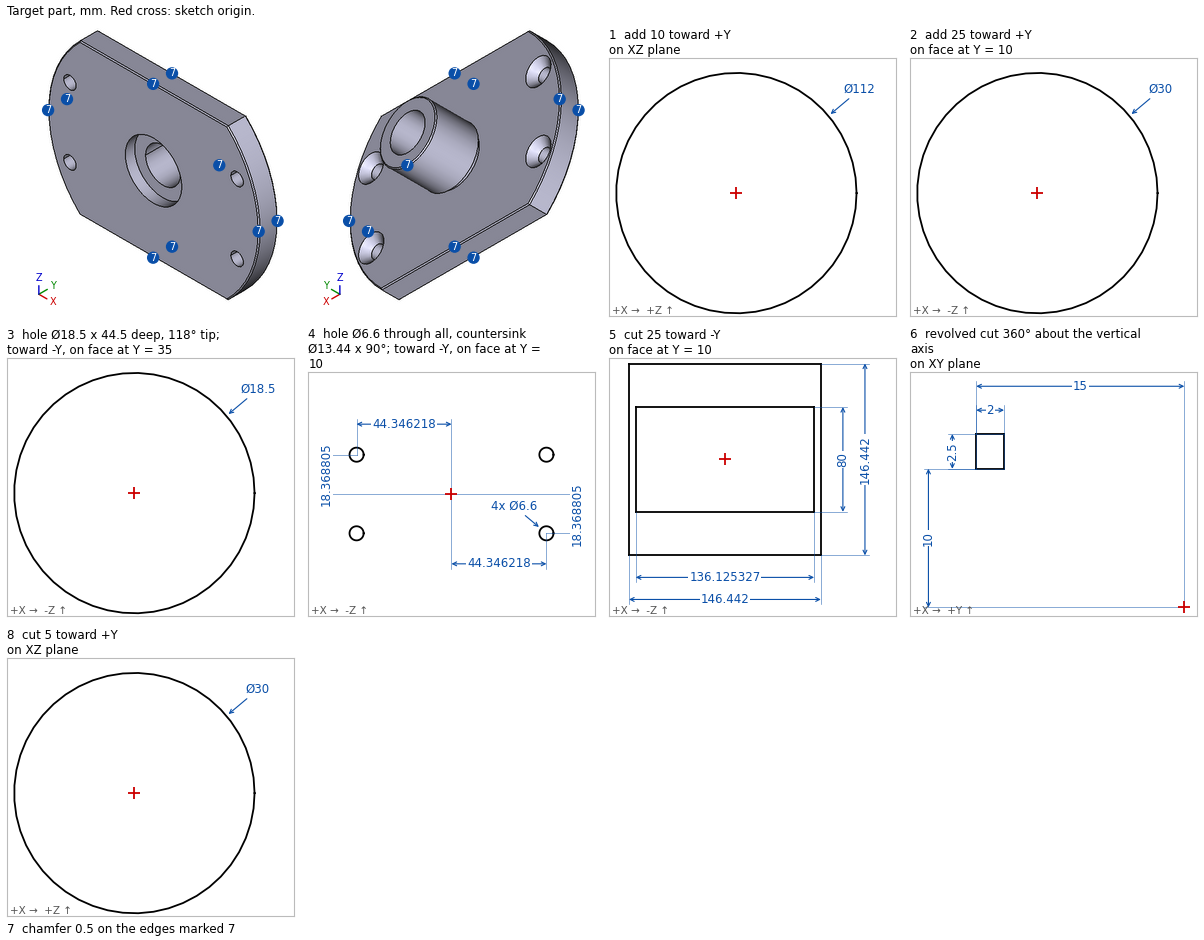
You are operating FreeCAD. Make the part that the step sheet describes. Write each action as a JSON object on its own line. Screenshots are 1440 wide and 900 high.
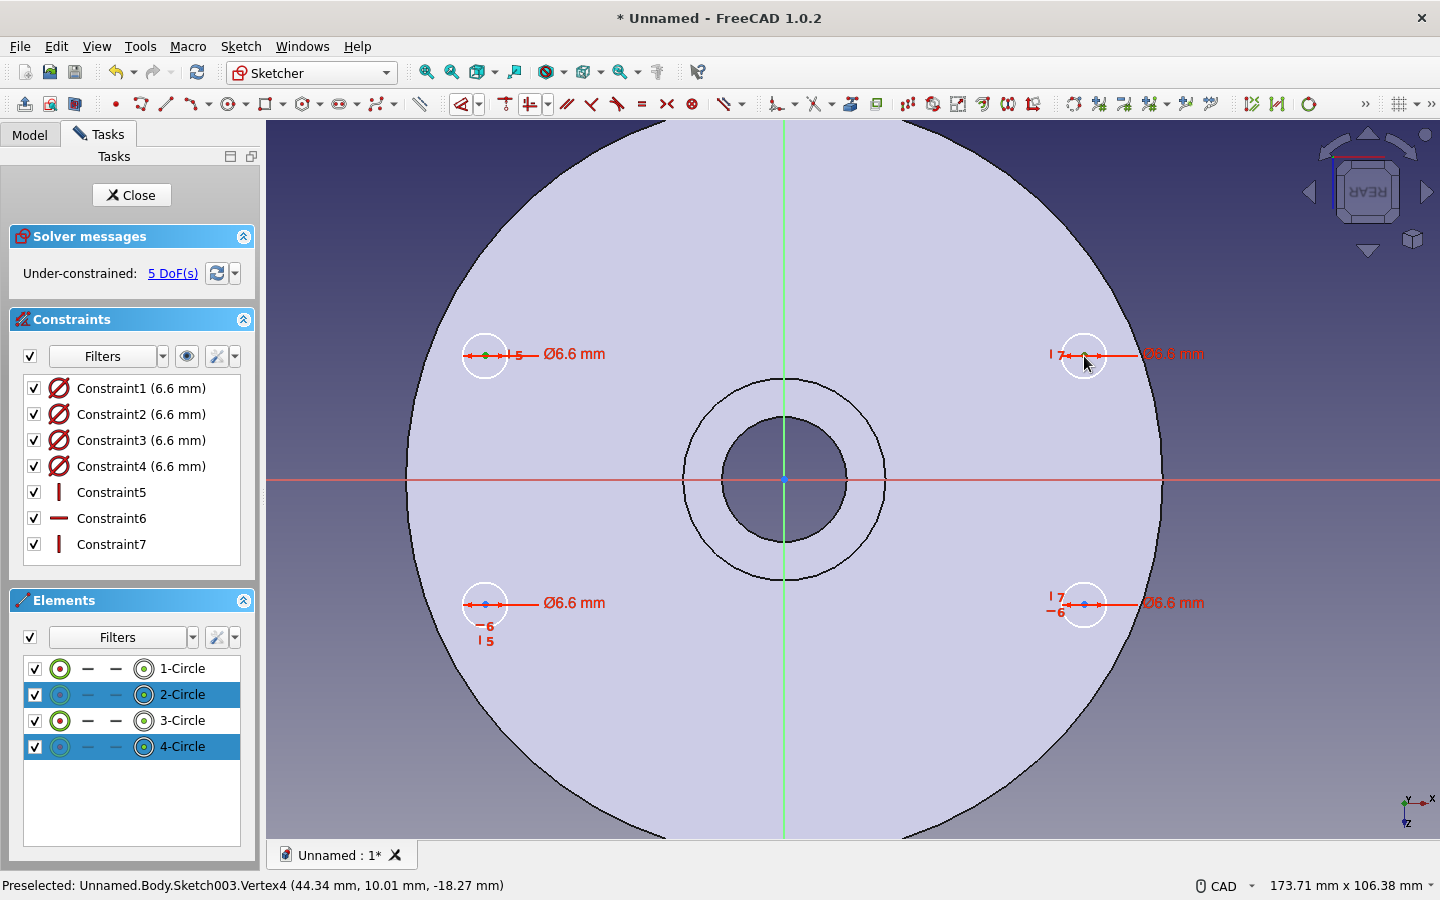
{"action": "key", "text": "h"}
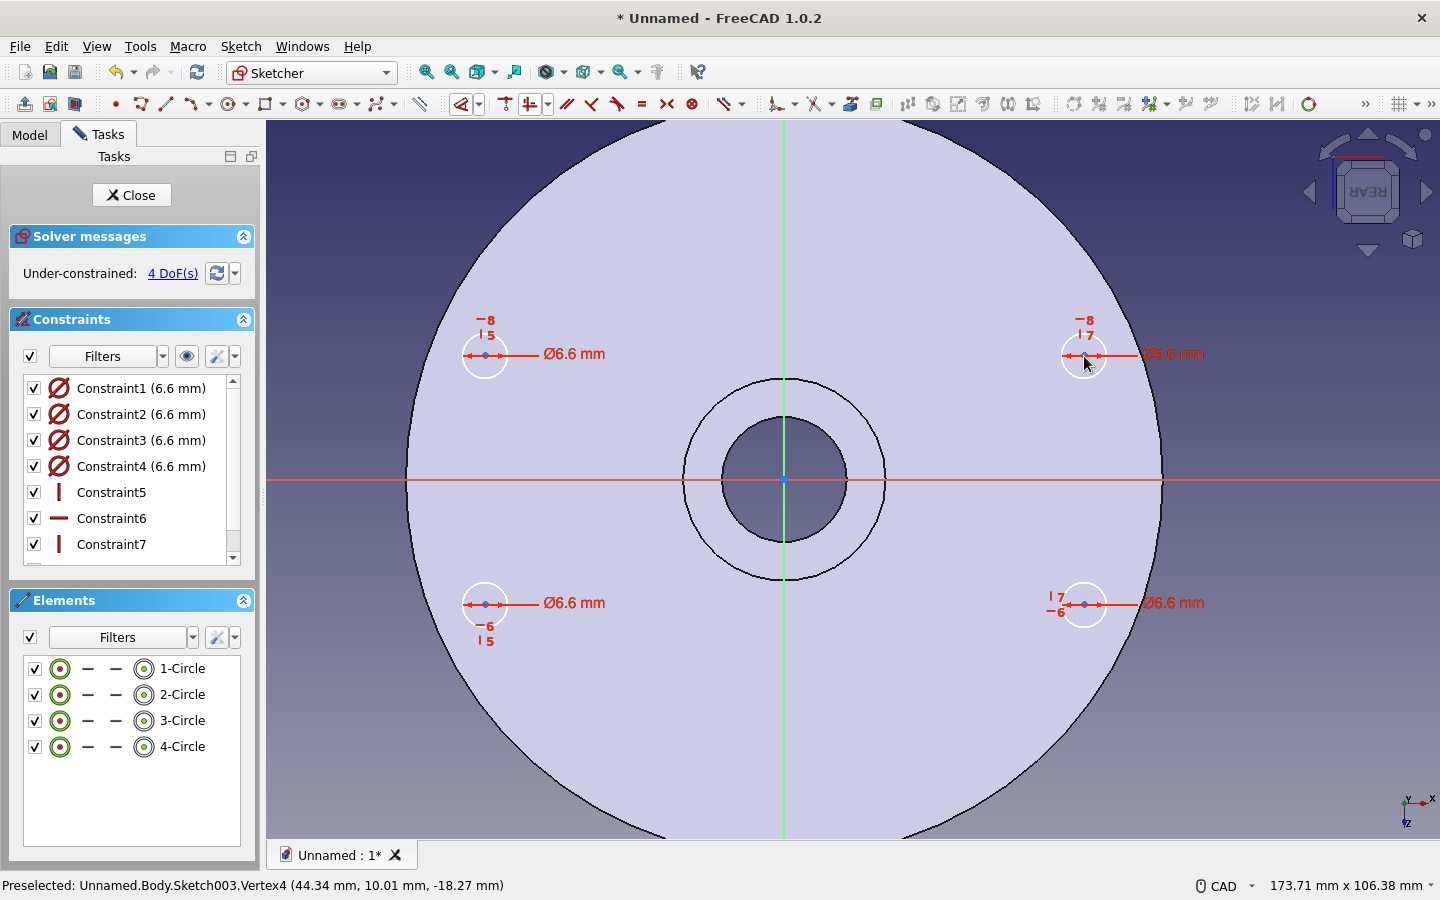
{"action": "left_click", "coordinate": [1084, 605]}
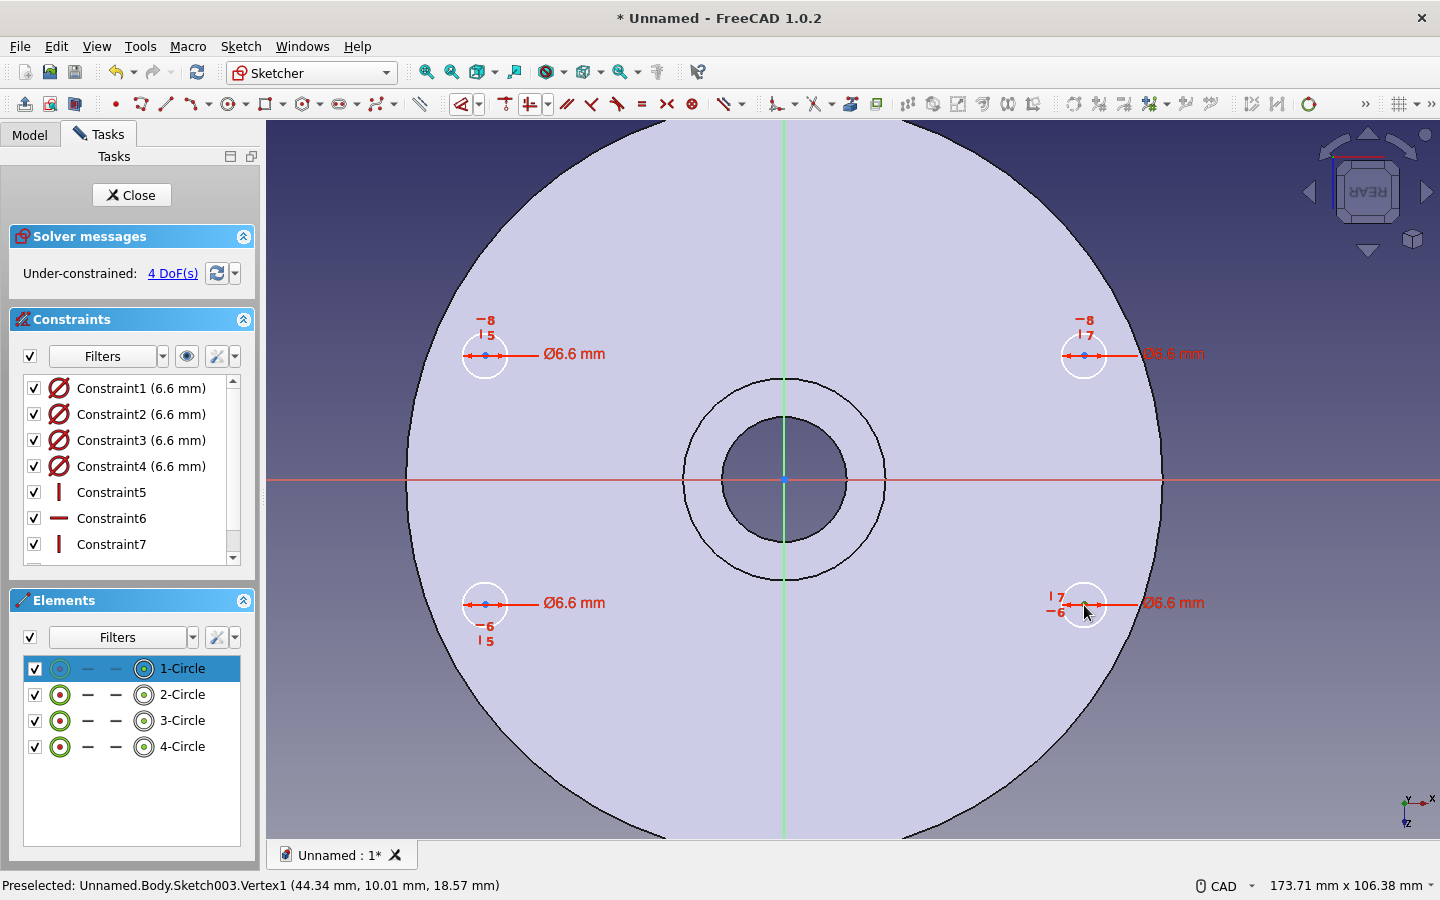
{"action": "key", "text": "l"}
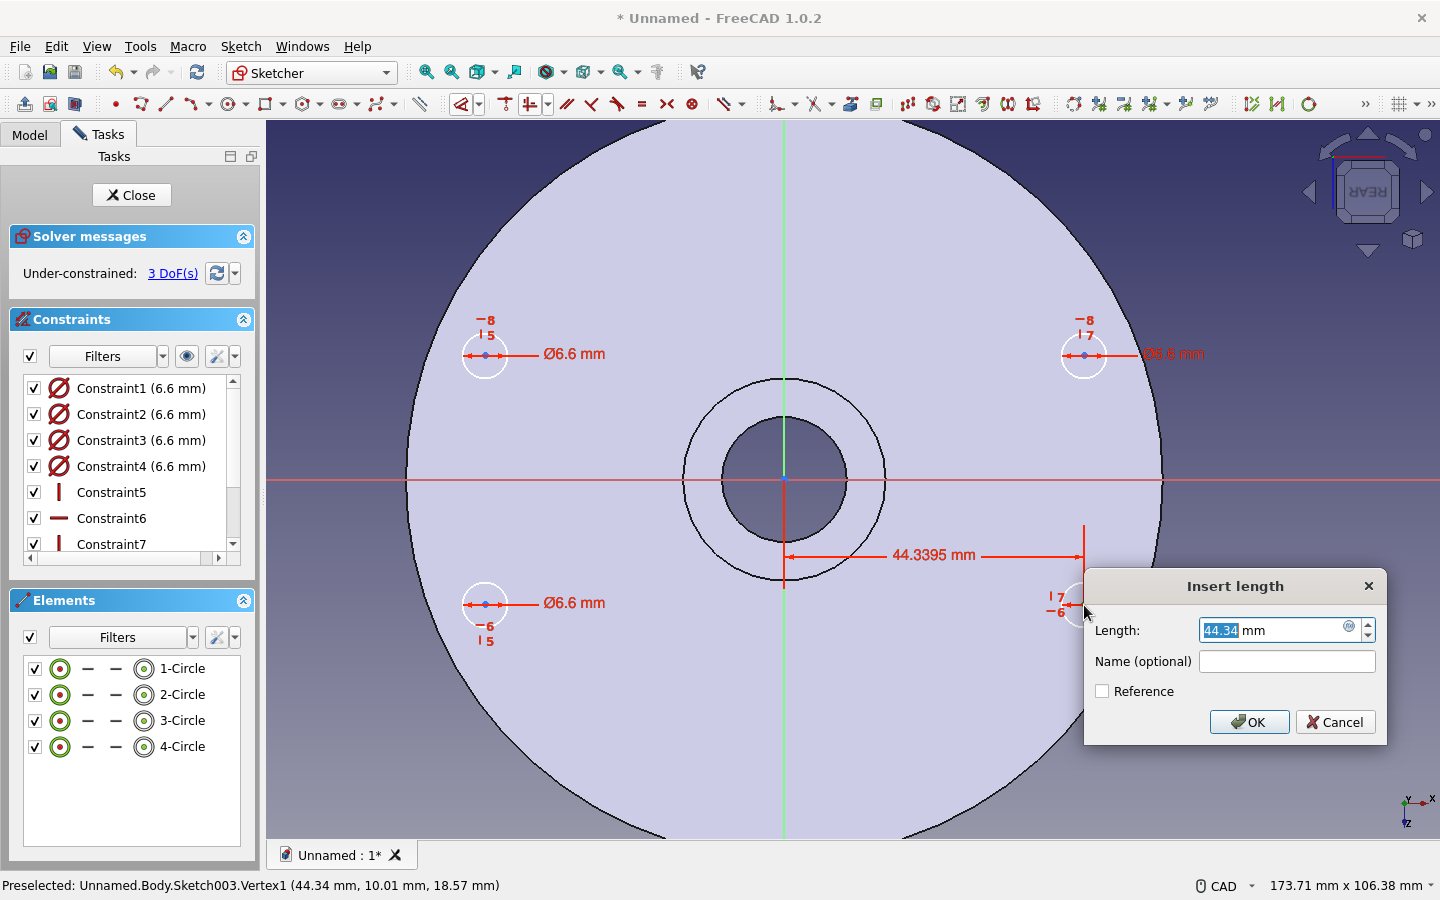
{"action": "type", "text": "44.346218"}
{"action": "key", "text": "Return"}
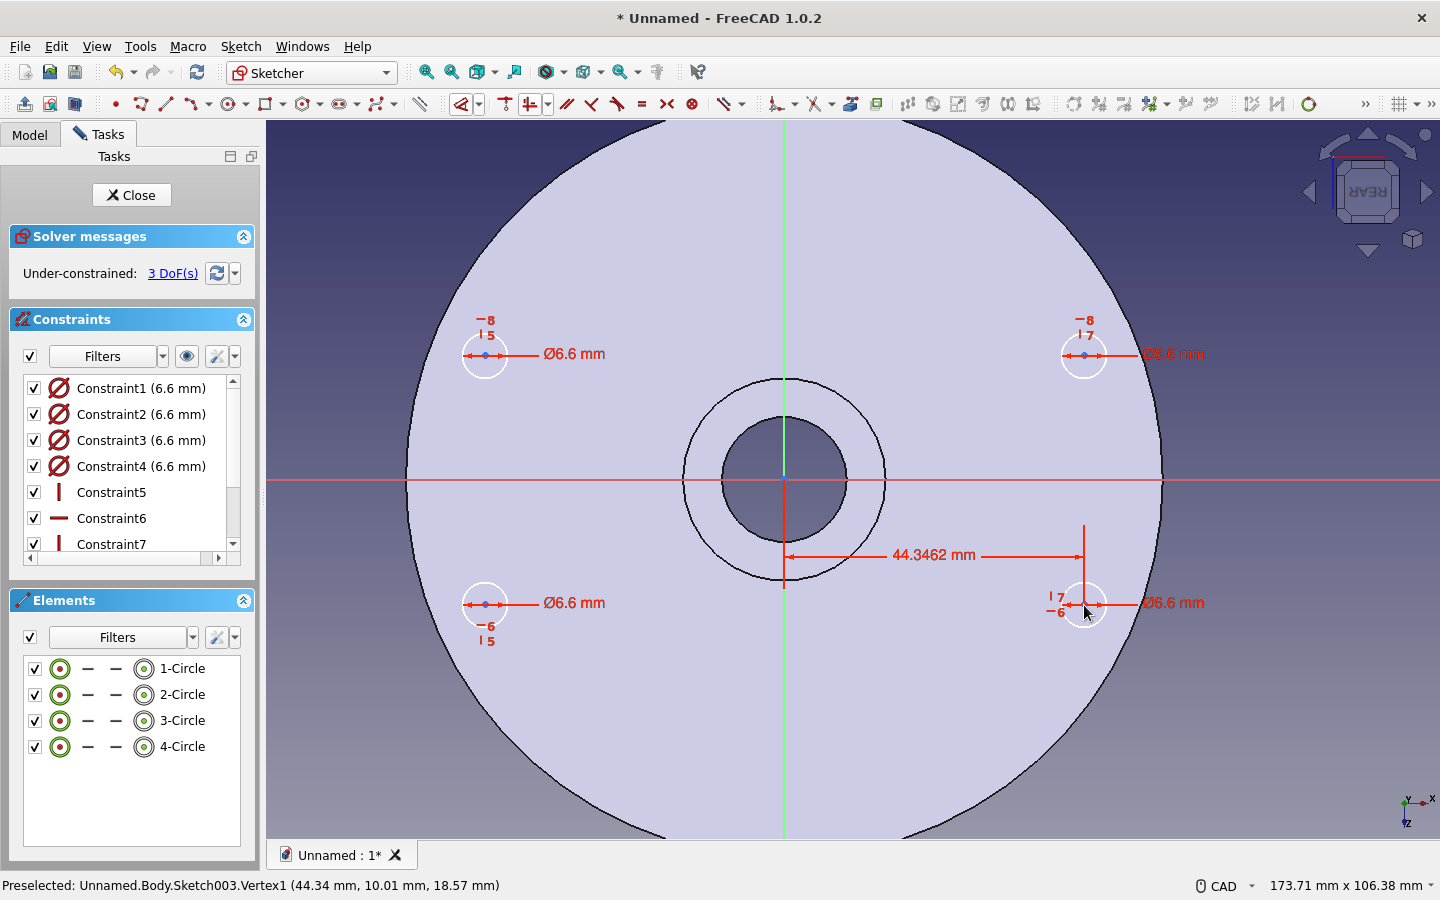
{"action": "left_click", "coordinate": [1084, 605]}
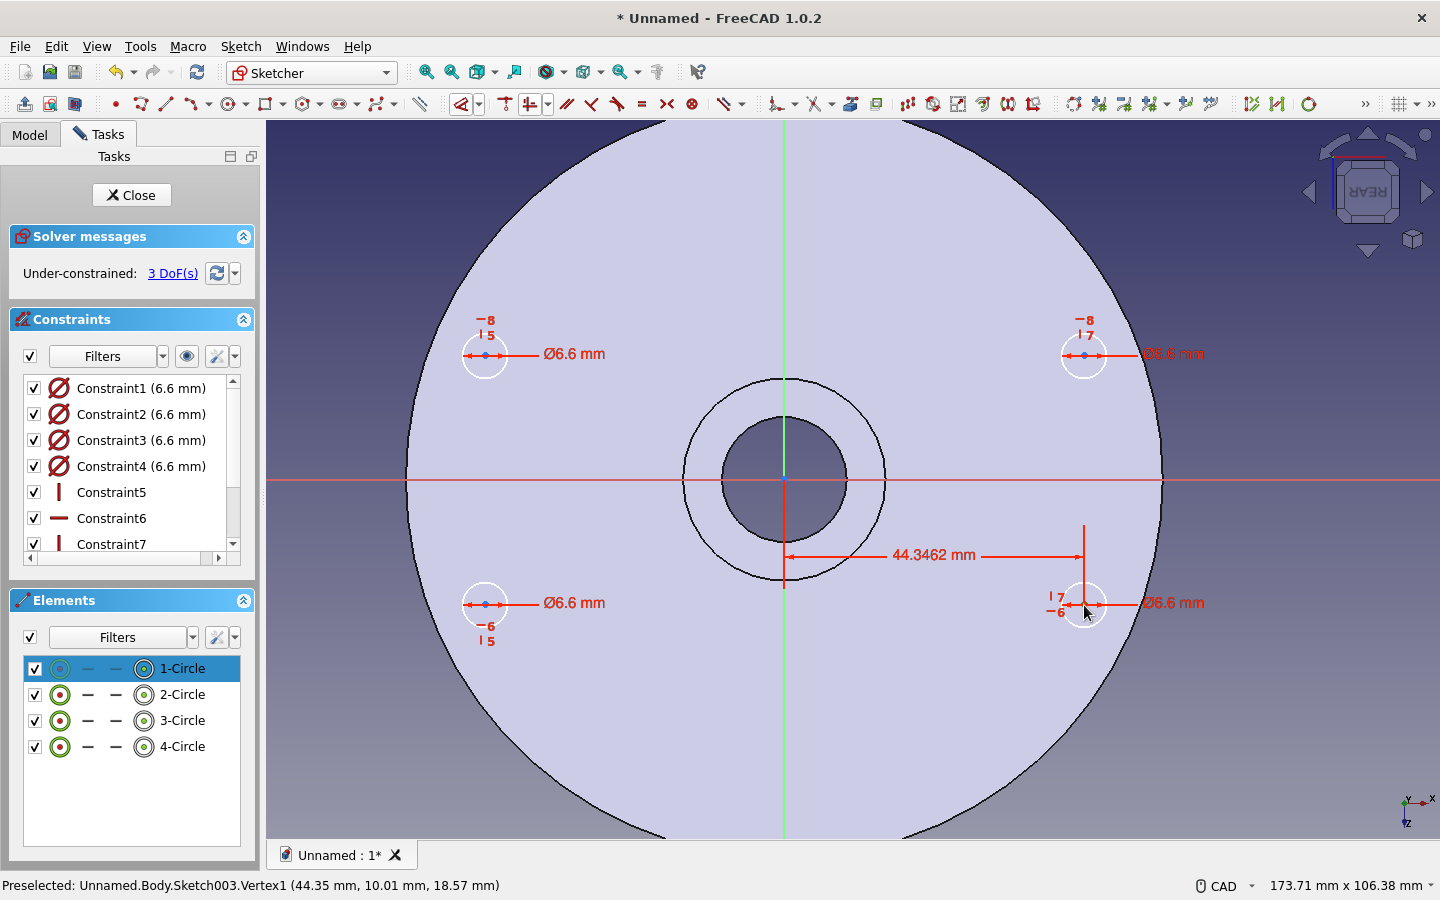
{"action": "key", "text": "i"}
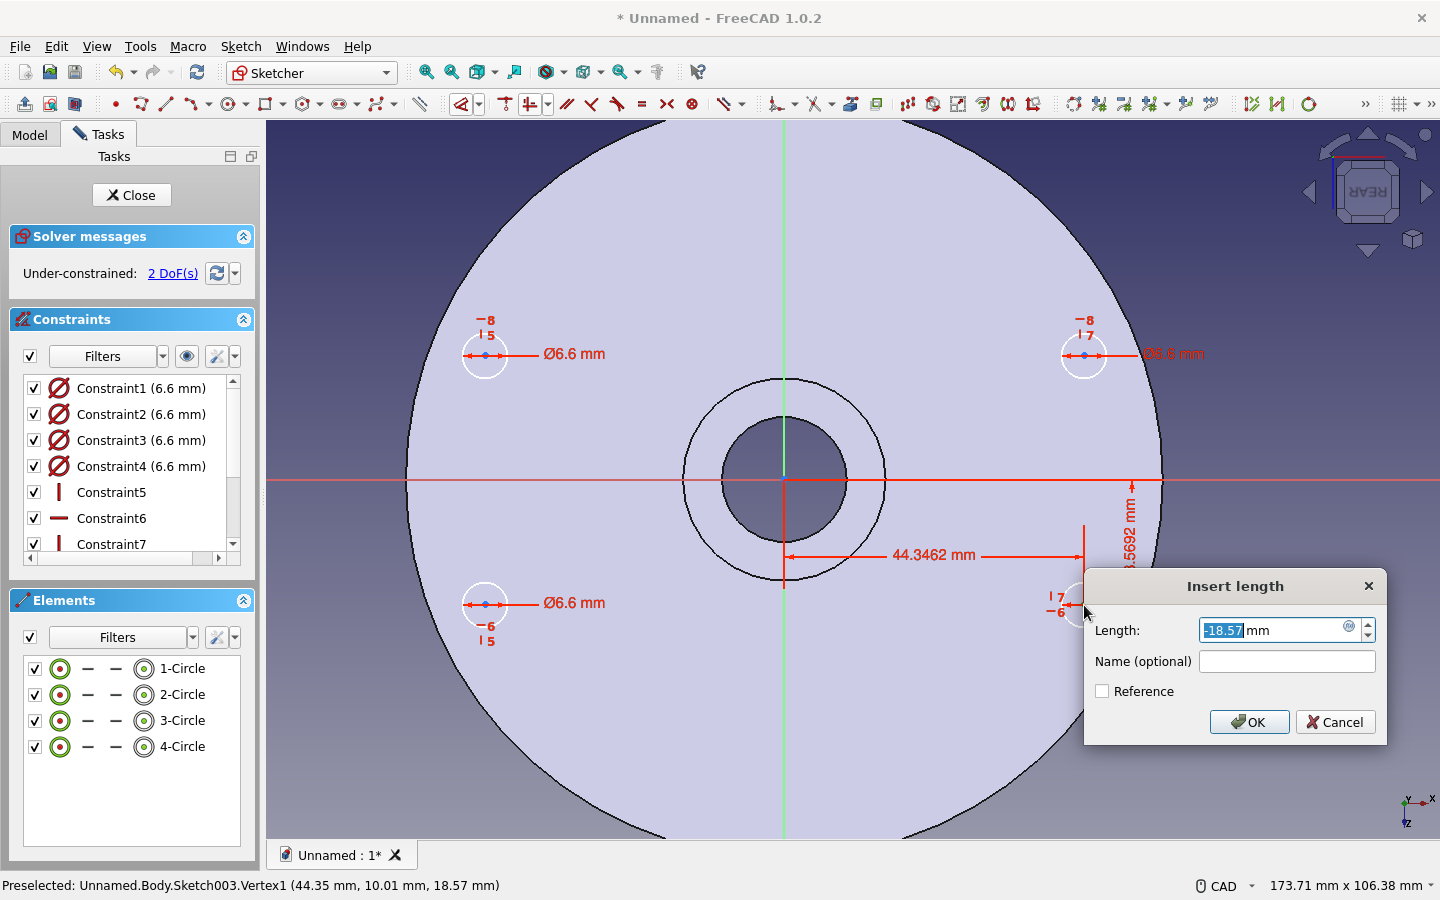
{"action": "type", "text": "-18.368805"}
{"action": "key", "text": "Return"}